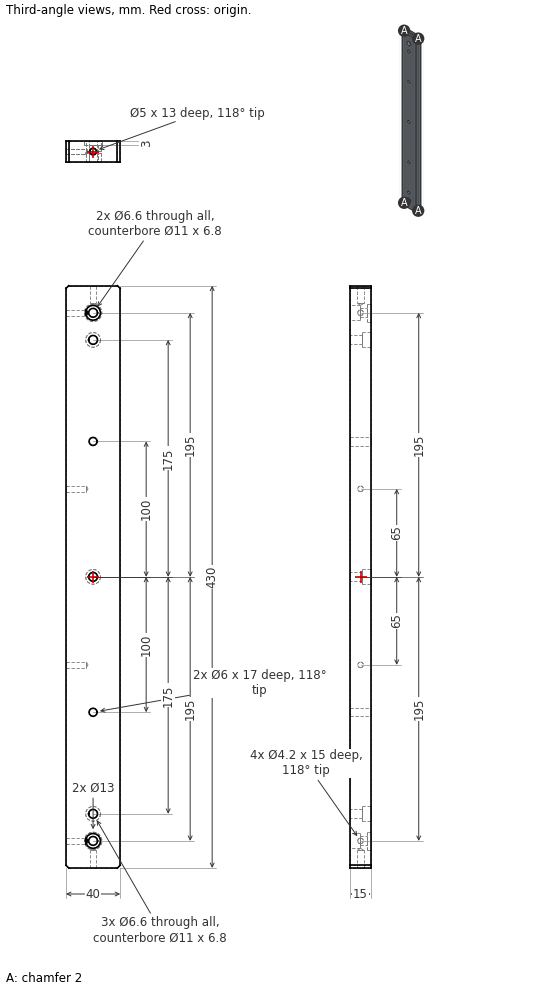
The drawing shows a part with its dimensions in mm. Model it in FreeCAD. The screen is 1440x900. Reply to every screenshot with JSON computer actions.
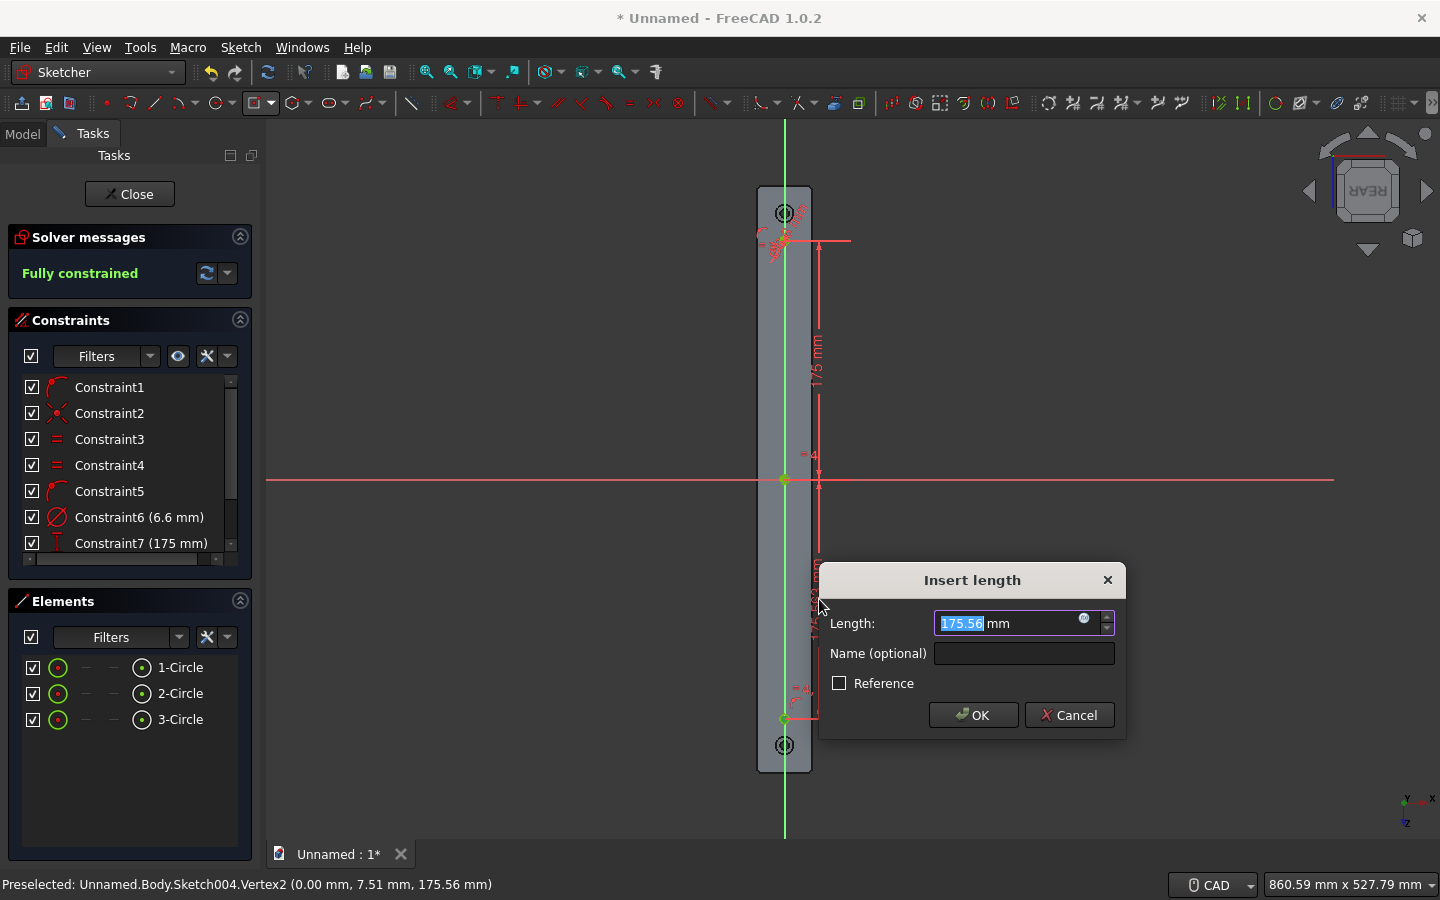
{"action": "type", "text": "175"}
{"action": "key", "text": "Return"}
{"action": "key", "text": "Escape"}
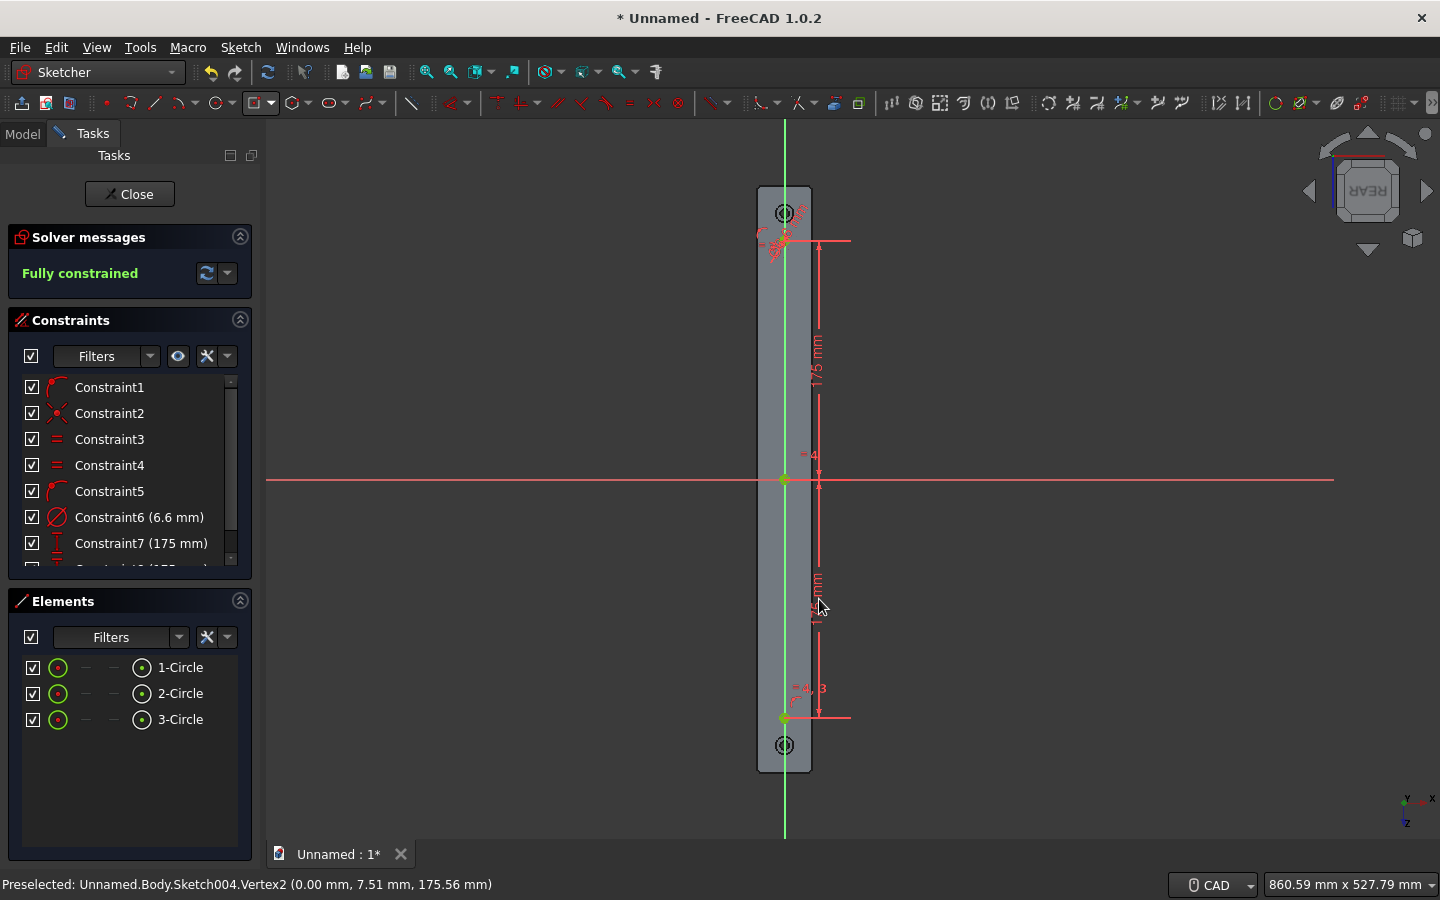
{"action": "left_click", "coordinate": [130, 194]}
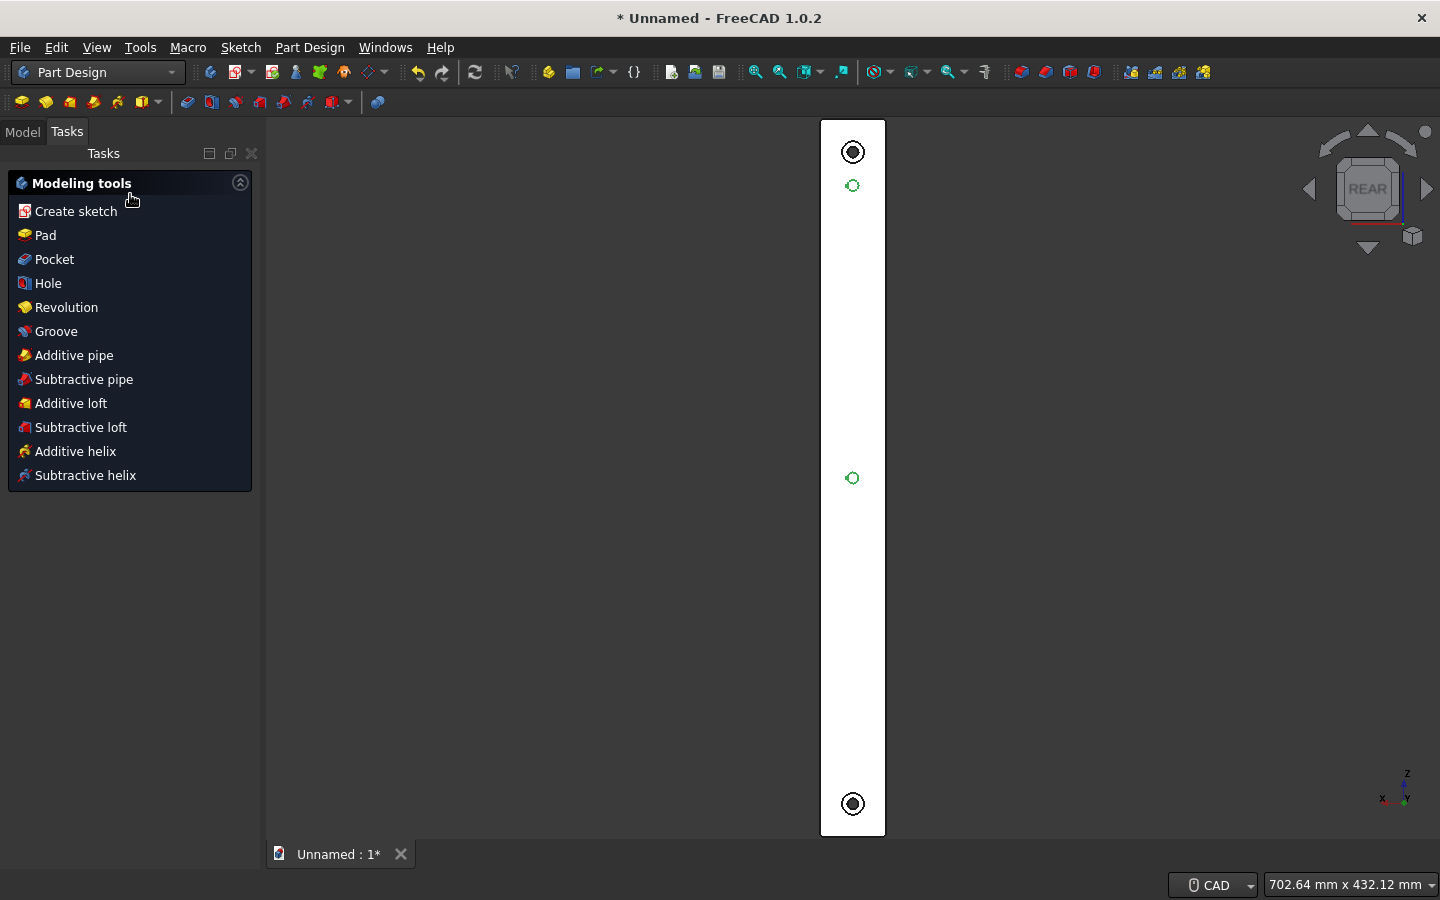
{"action": "left_click", "coordinate": [212, 102]}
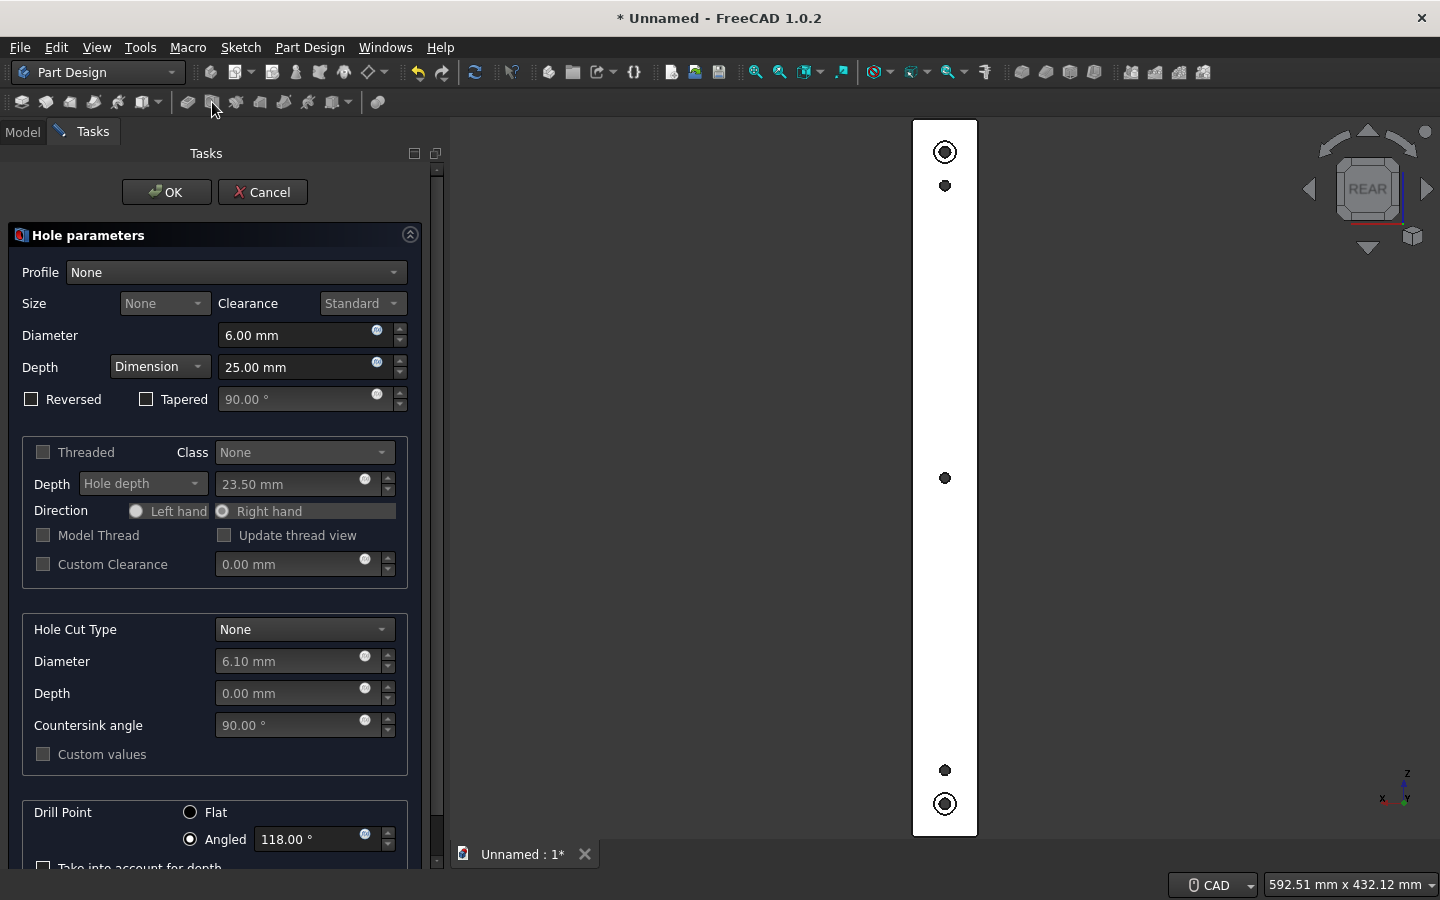
{"action": "triple_click", "coordinate": [305, 335]}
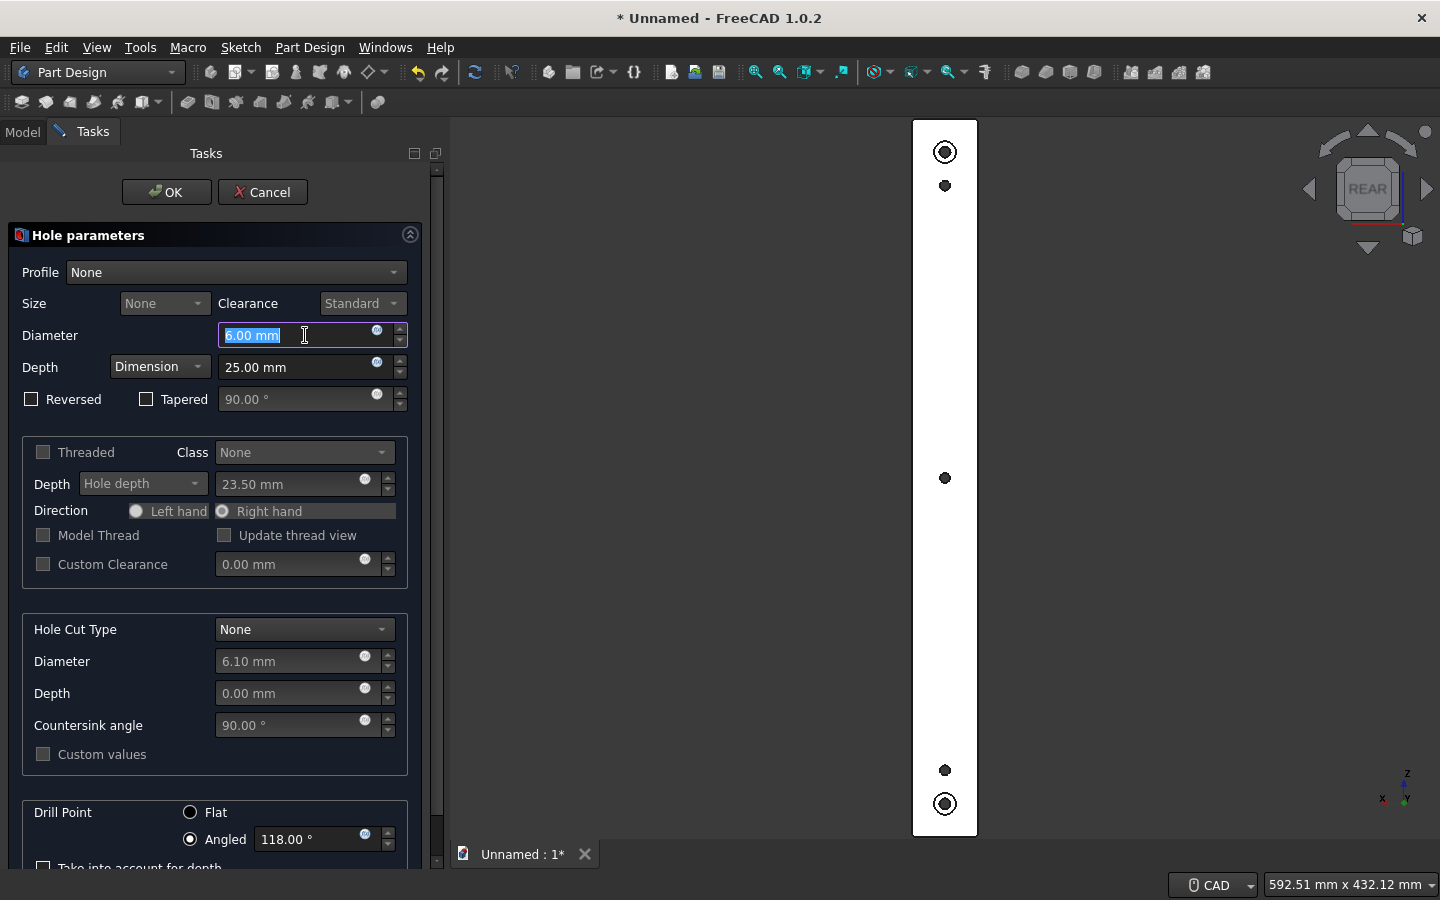
{"action": "type", "text": "6.6"}
{"action": "key", "text": "Tab"}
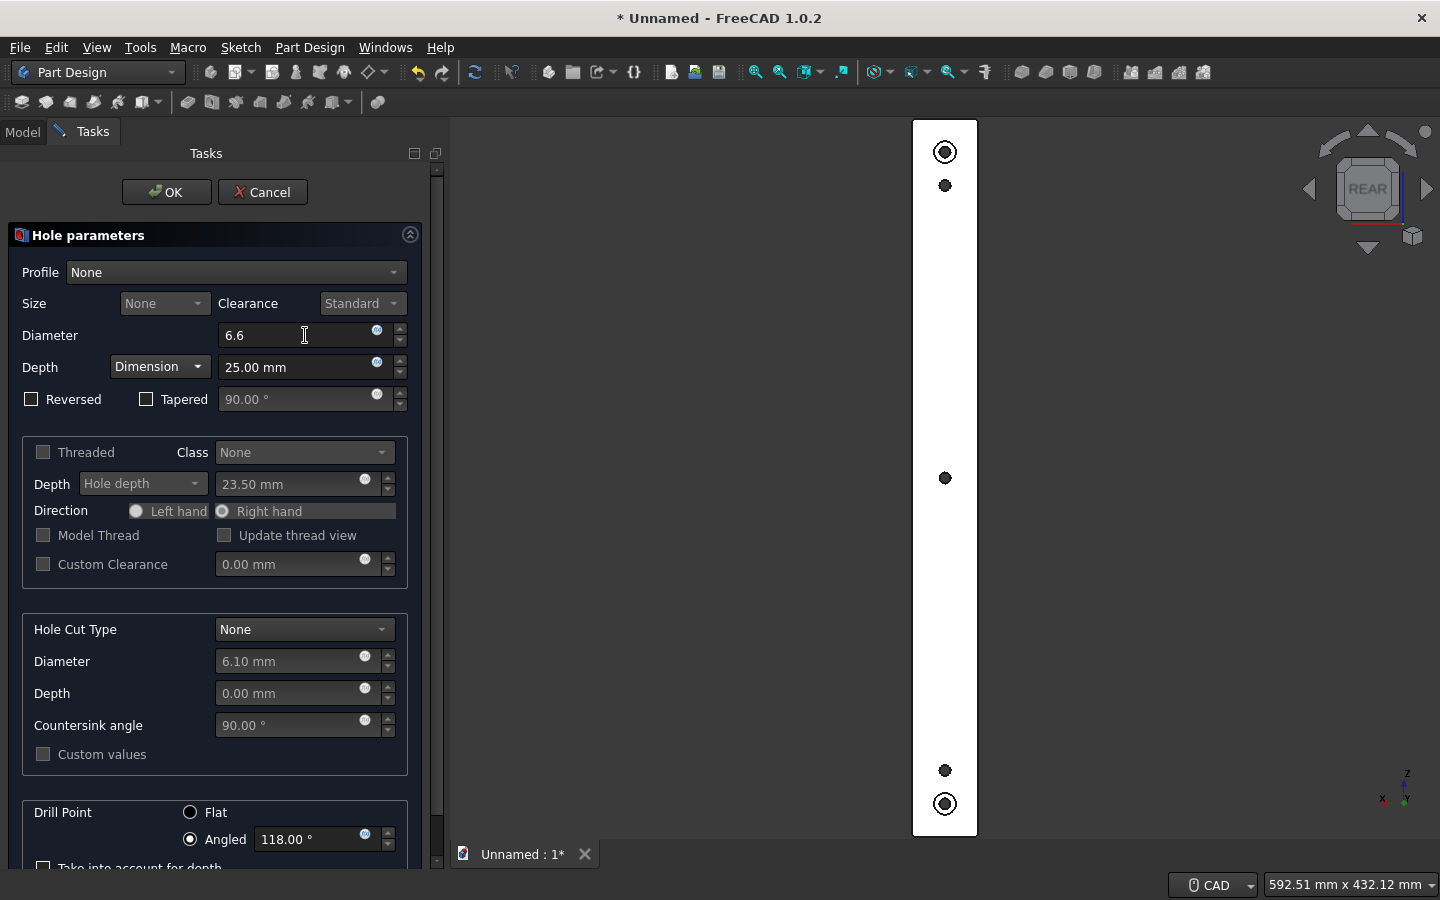
{"action": "left_click", "coordinate": [161, 366]}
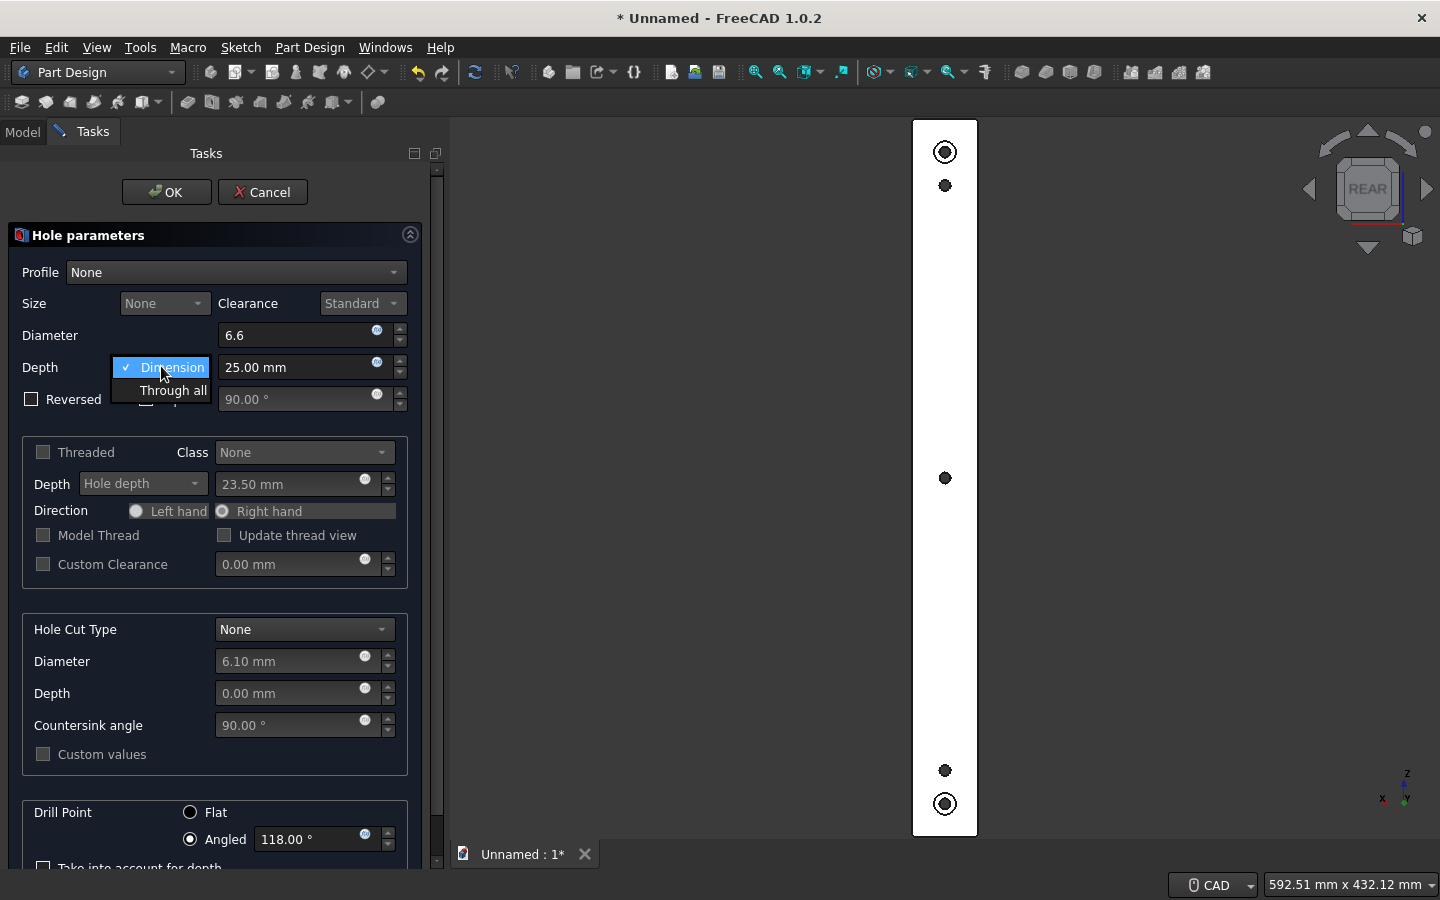
{"action": "left_click", "coordinate": [160, 390]}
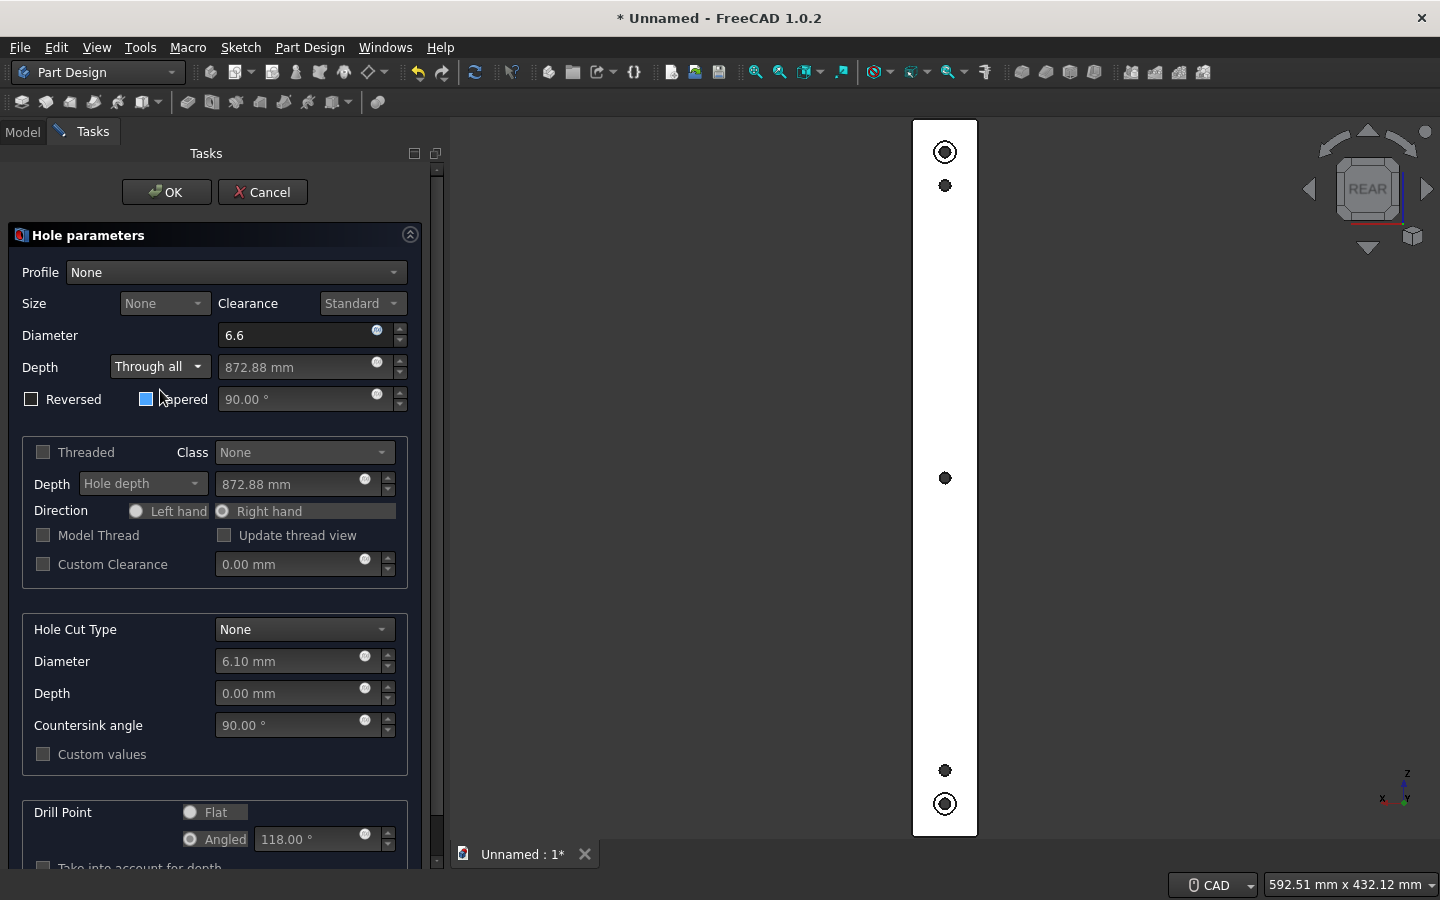
{"action": "left_click", "coordinate": [306, 630]}